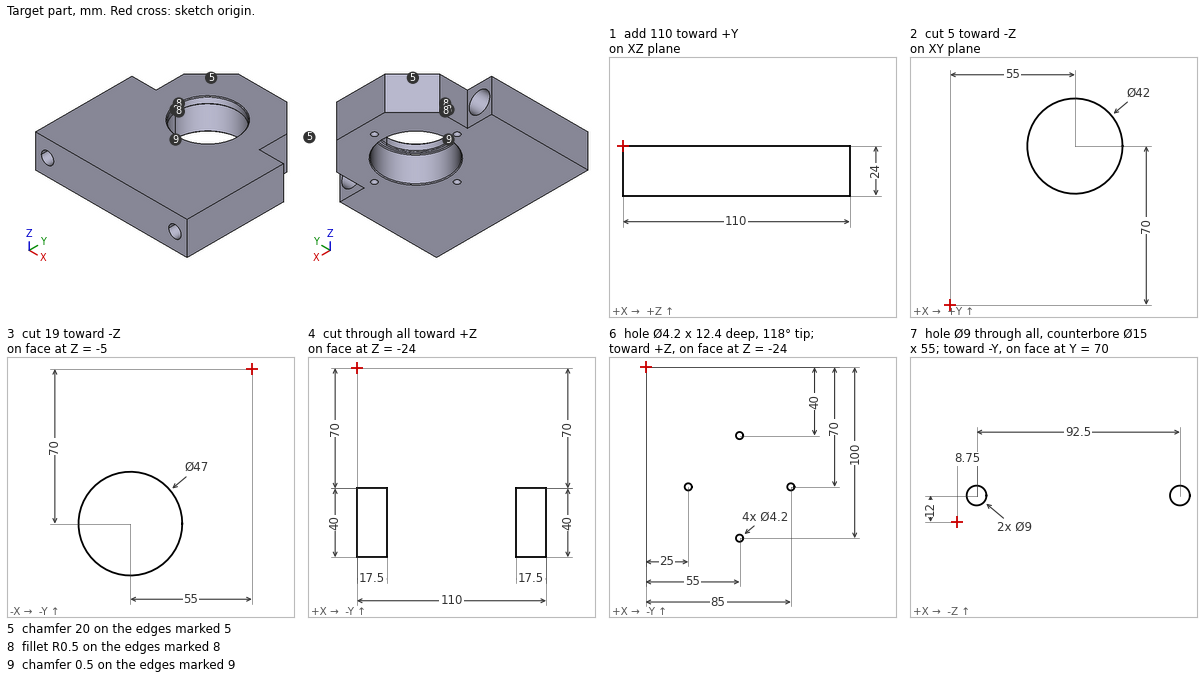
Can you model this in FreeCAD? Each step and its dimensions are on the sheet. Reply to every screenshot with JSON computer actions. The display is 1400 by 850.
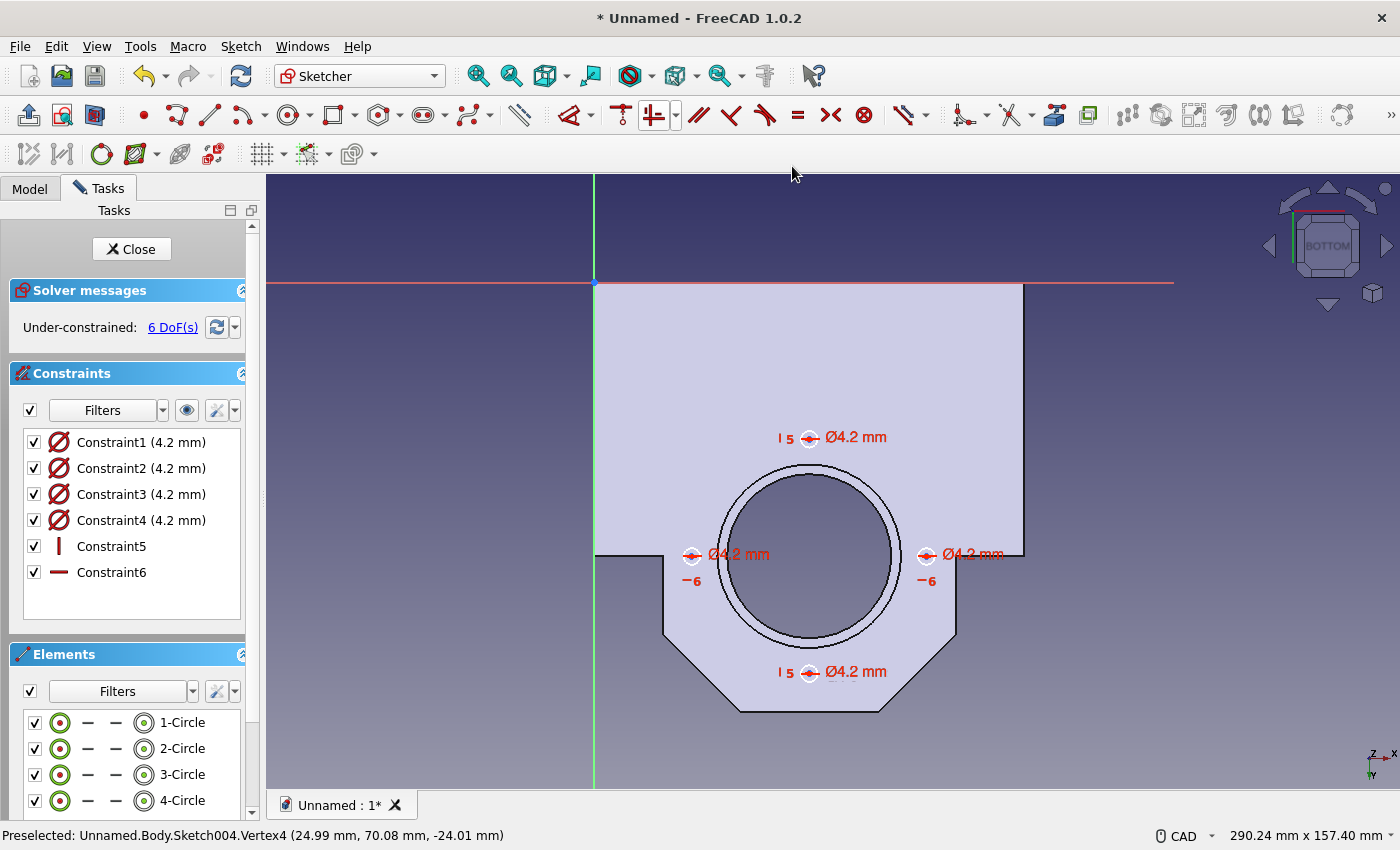
{"action": "key", "text": "d"}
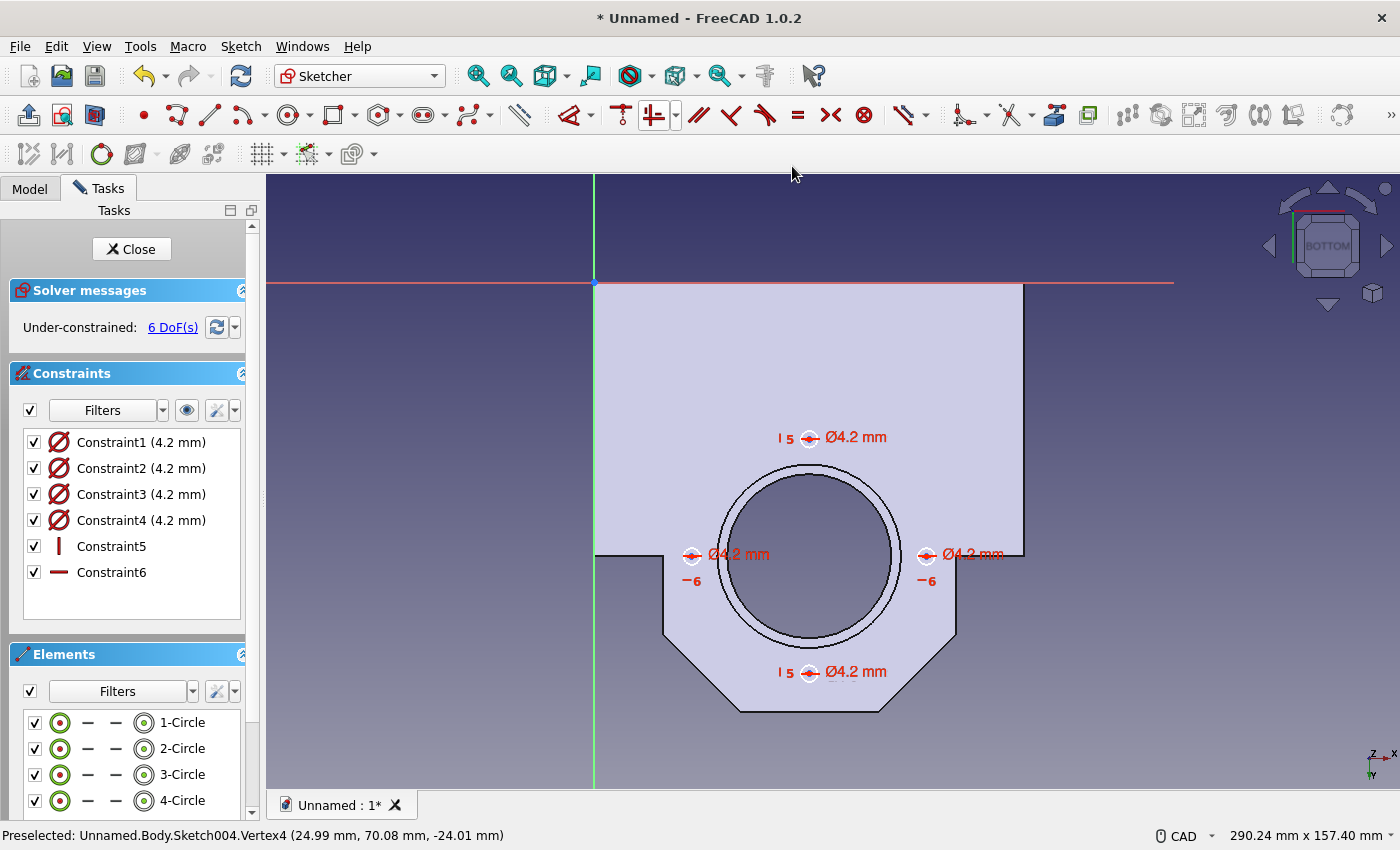
{"action": "left_click", "coordinate": [809, 674]}
{"action": "left_click", "coordinate": [702, 249]}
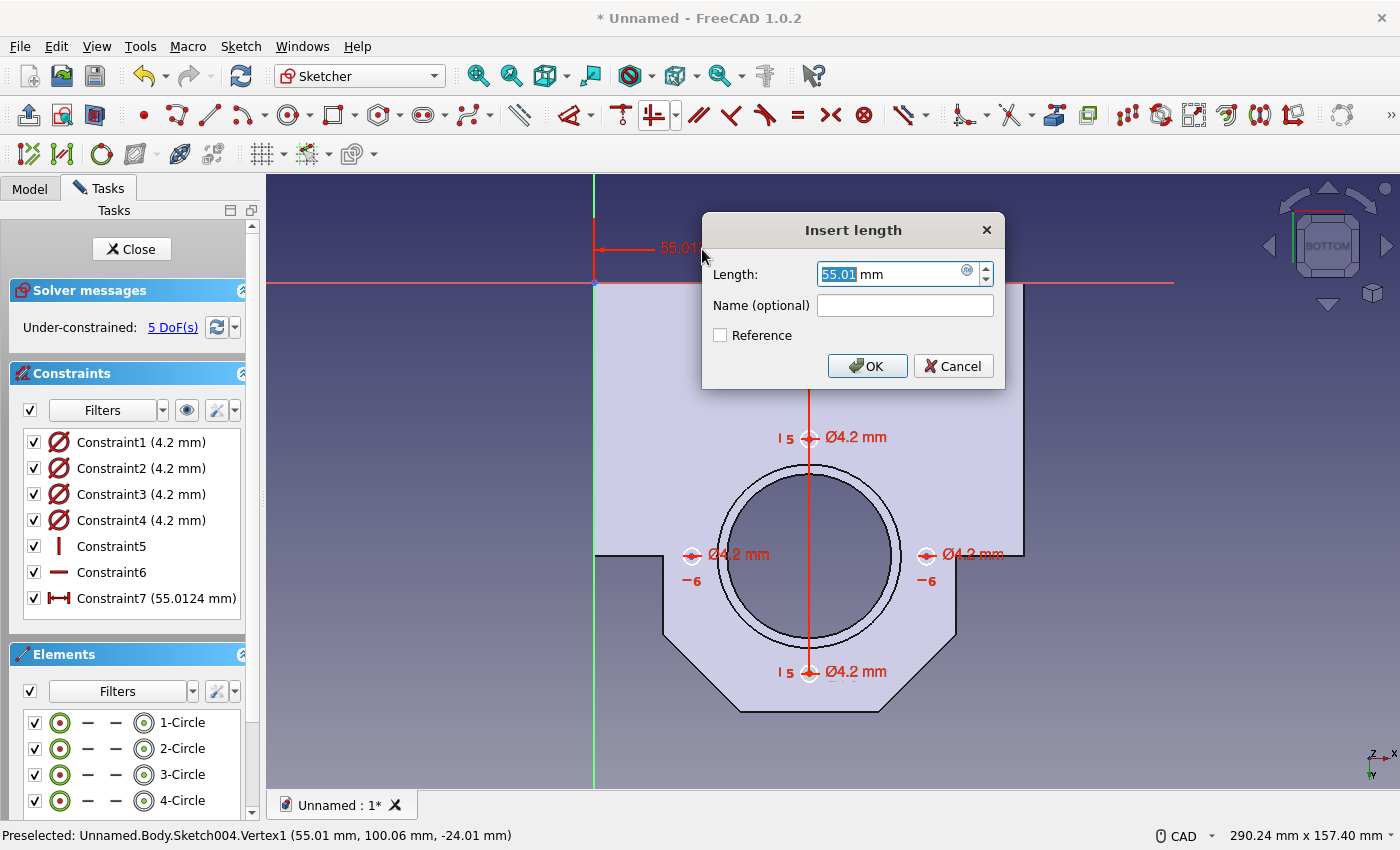
{"action": "type", "text": "55"}
{"action": "key", "text": "Return"}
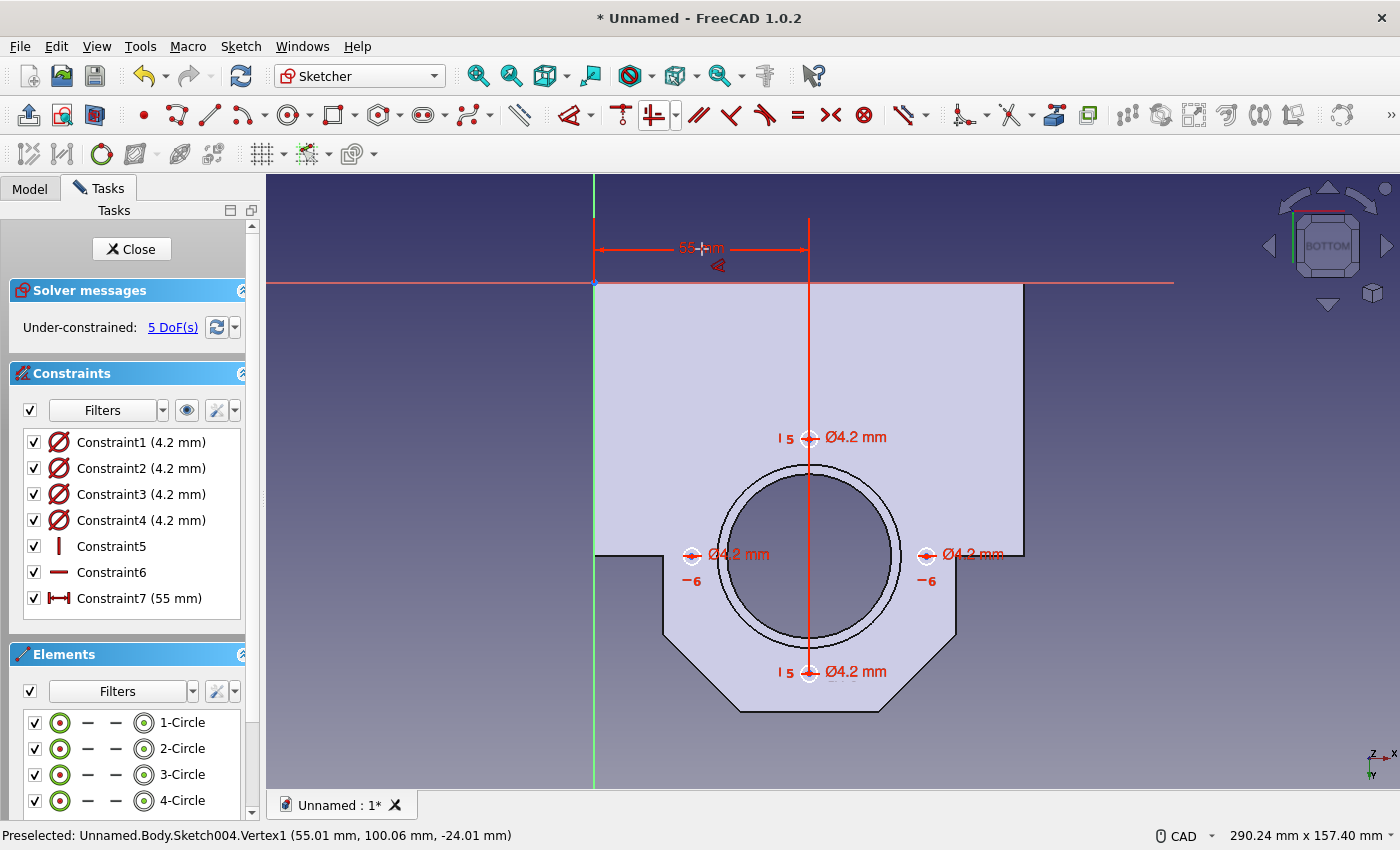
{"action": "left_click", "coordinate": [926, 556]}
{"action": "left_click", "coordinate": [837, 249]}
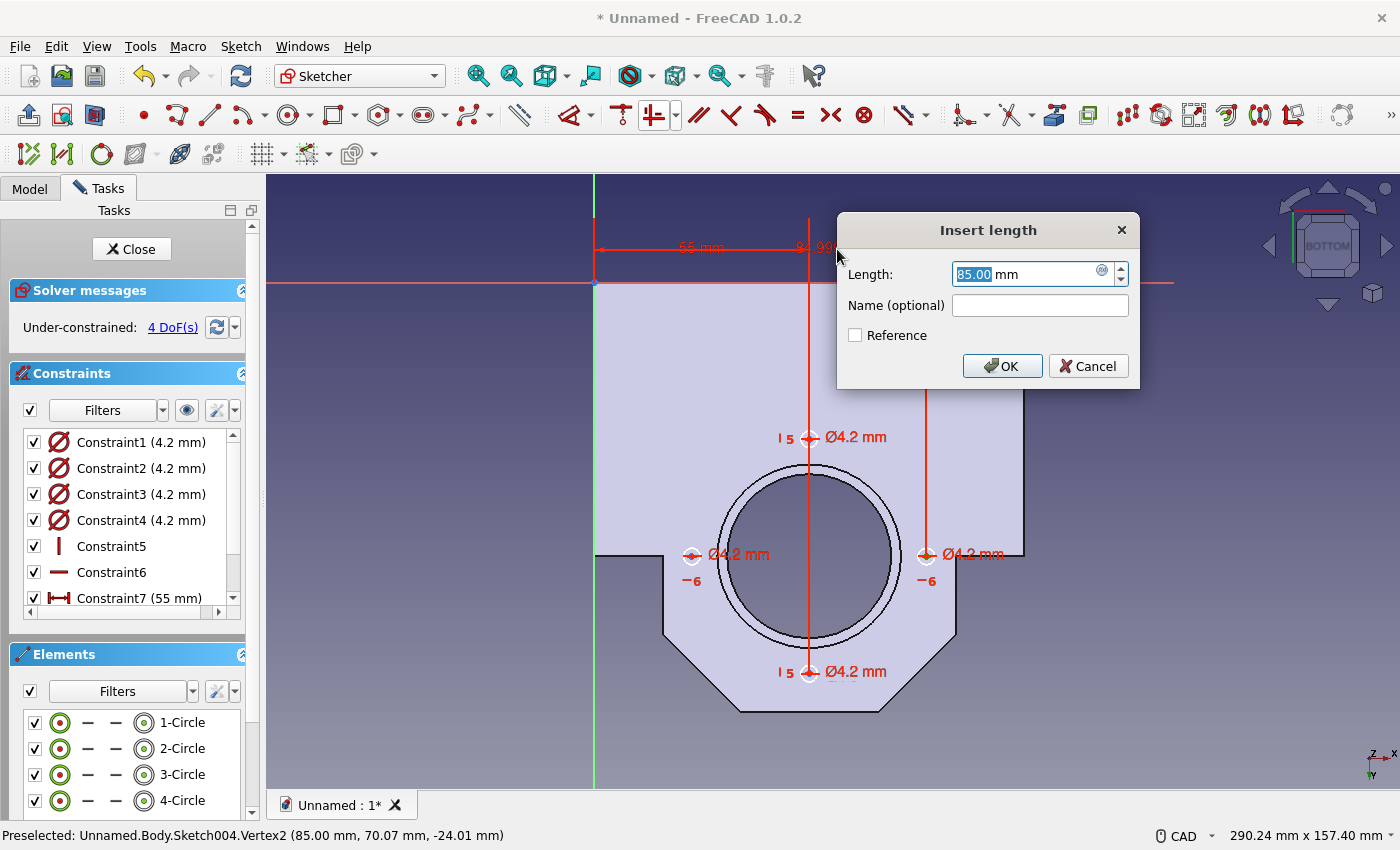
{"action": "type", "text": "85"}
{"action": "key", "text": "Return"}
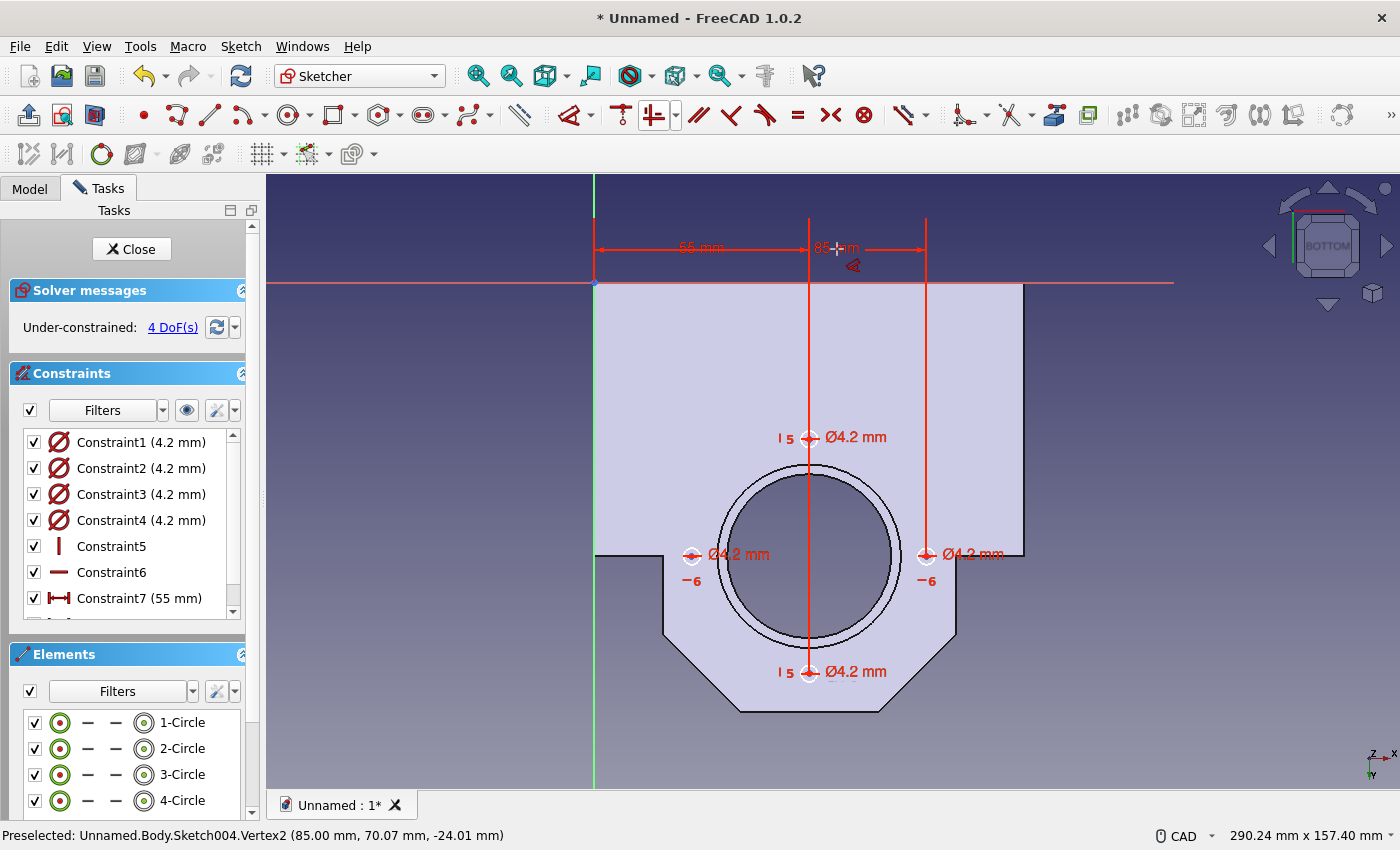
{"action": "left_click", "coordinate": [926, 556]}
{"action": "left_click", "coordinate": [560, 420]}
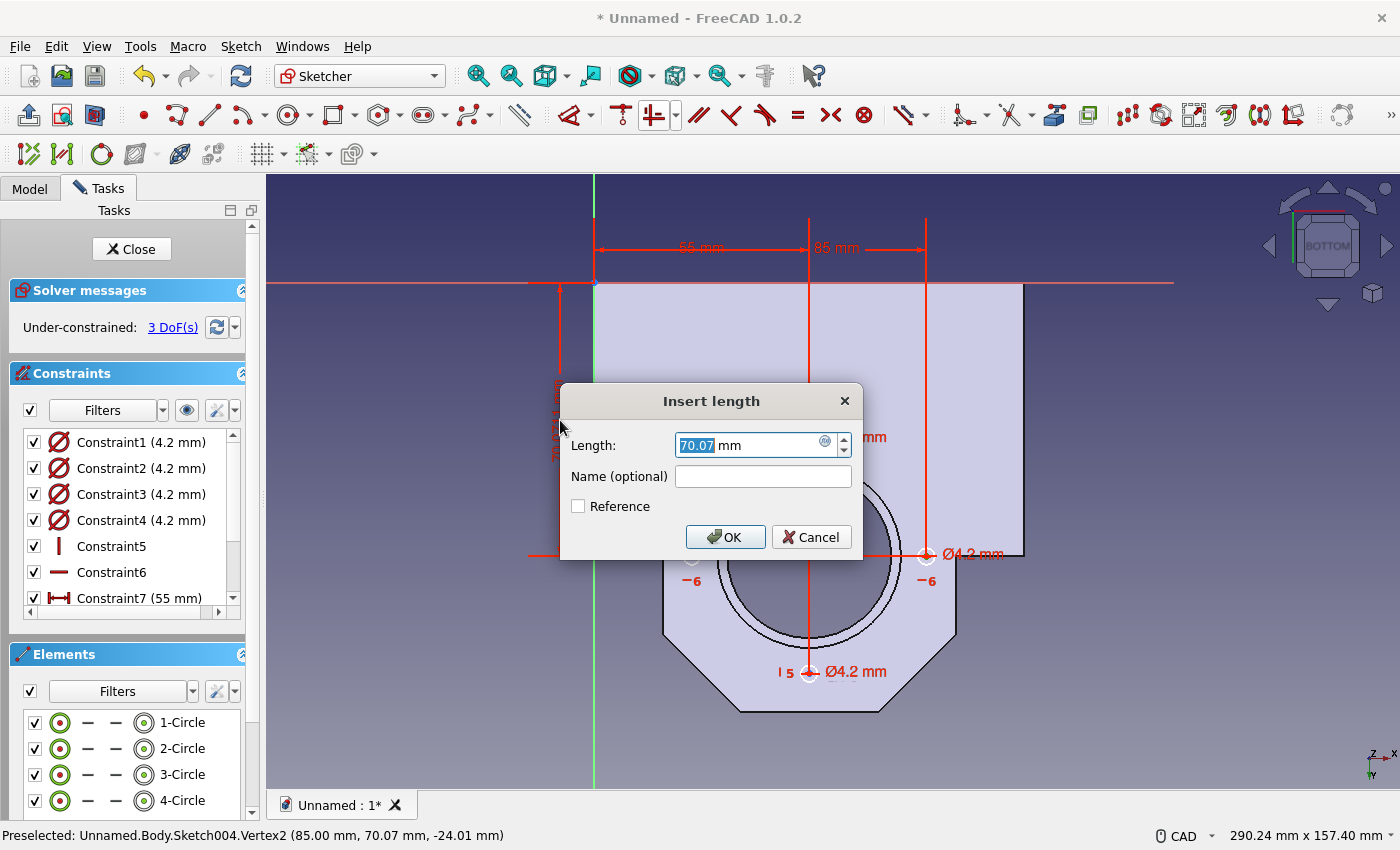
{"action": "type", "text": "70"}
{"action": "key", "text": "Return"}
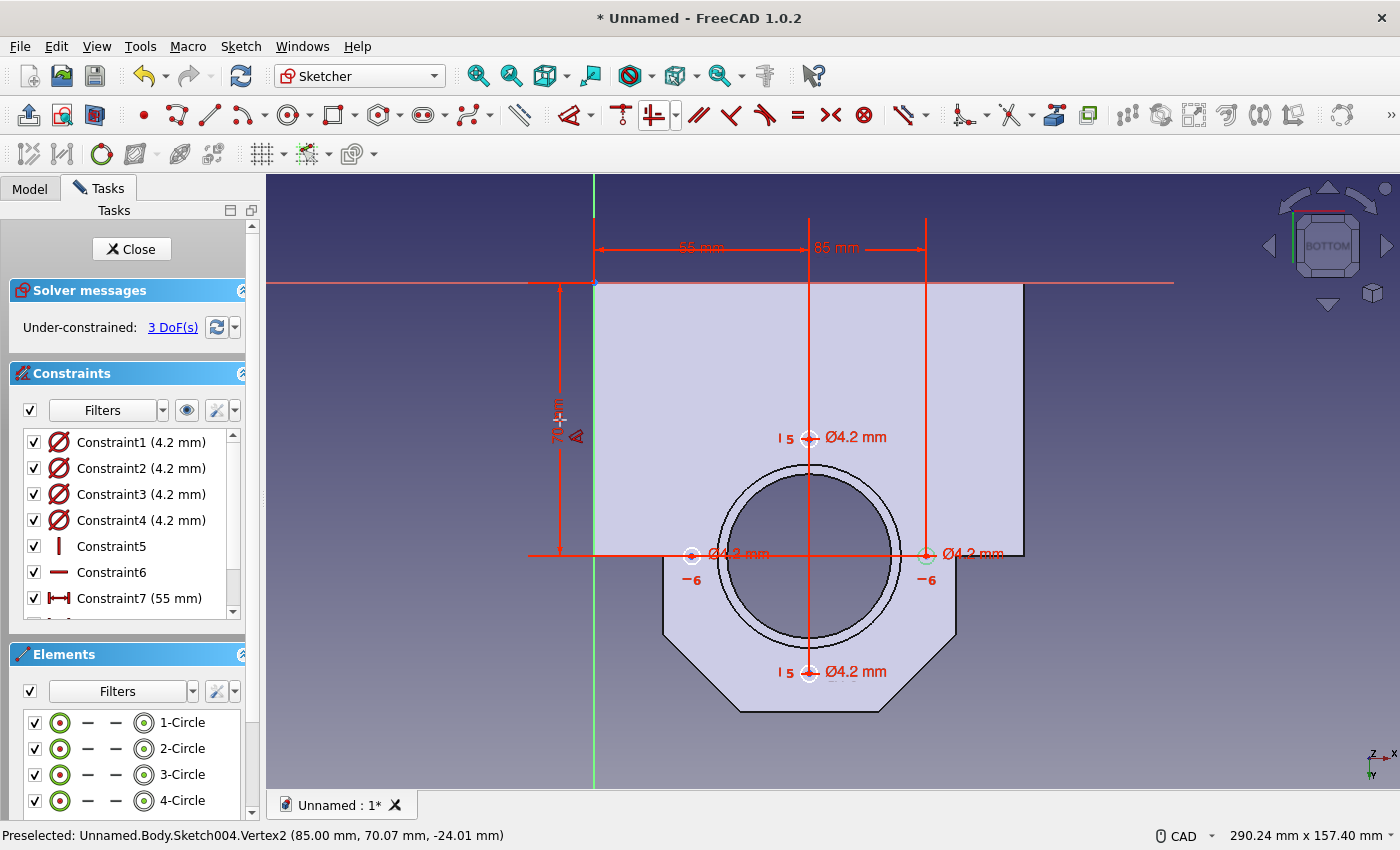
{"action": "left_click", "coordinate": [809, 439]}
{"action": "left_click", "coordinate": [560, 361]}